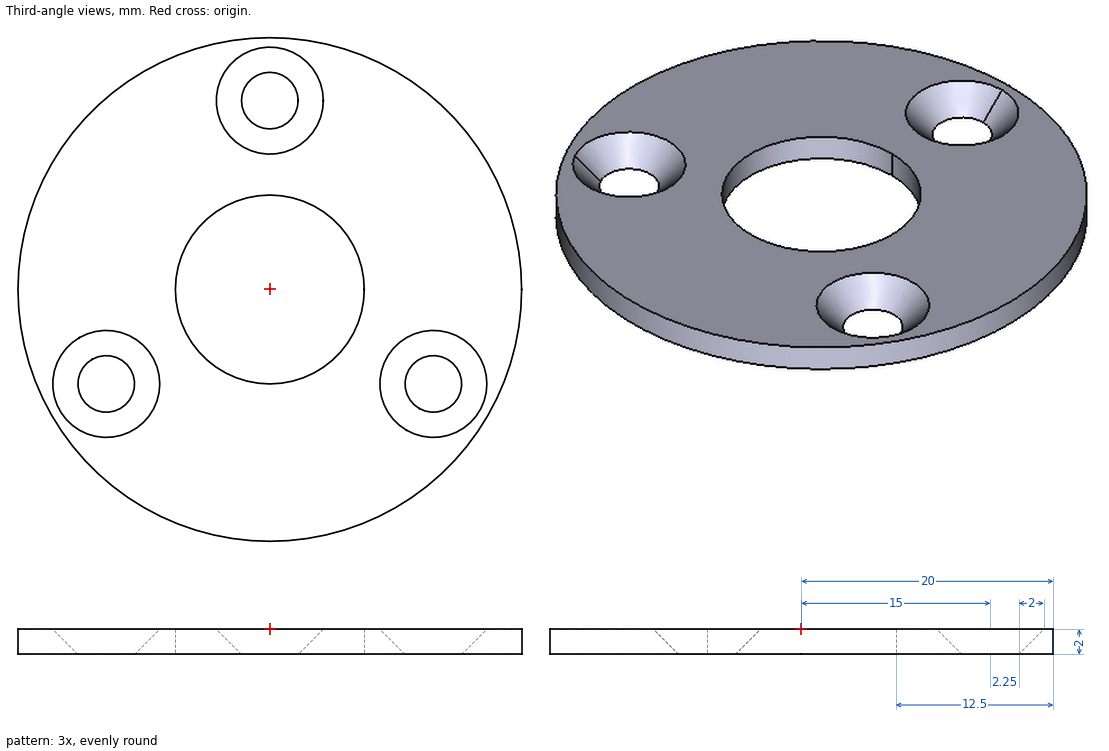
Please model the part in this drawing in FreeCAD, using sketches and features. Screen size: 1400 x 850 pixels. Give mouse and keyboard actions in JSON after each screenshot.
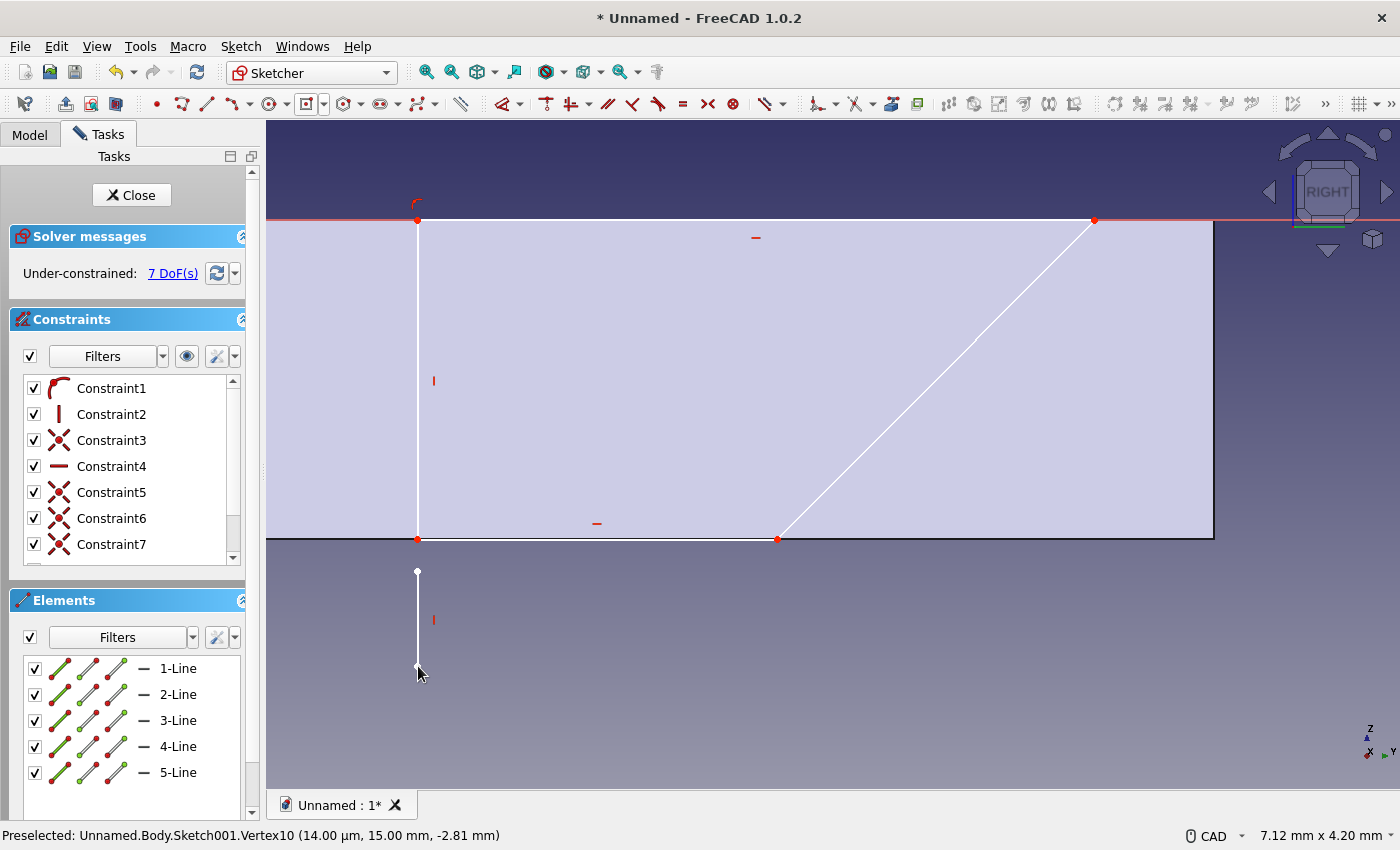
{"action": "left_click", "coordinate": [418, 601]}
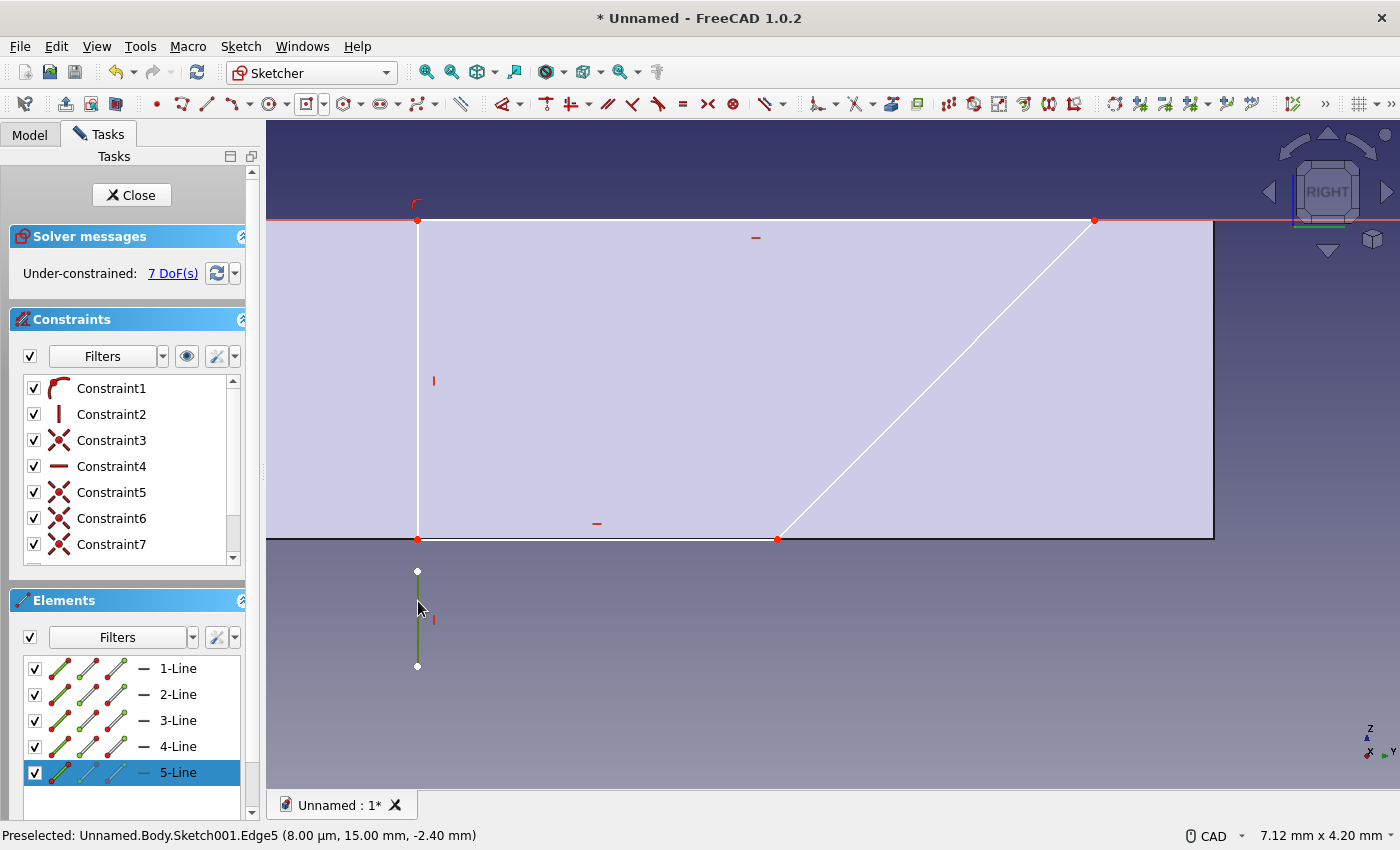
{"action": "left_click", "coordinate": [461, 104]}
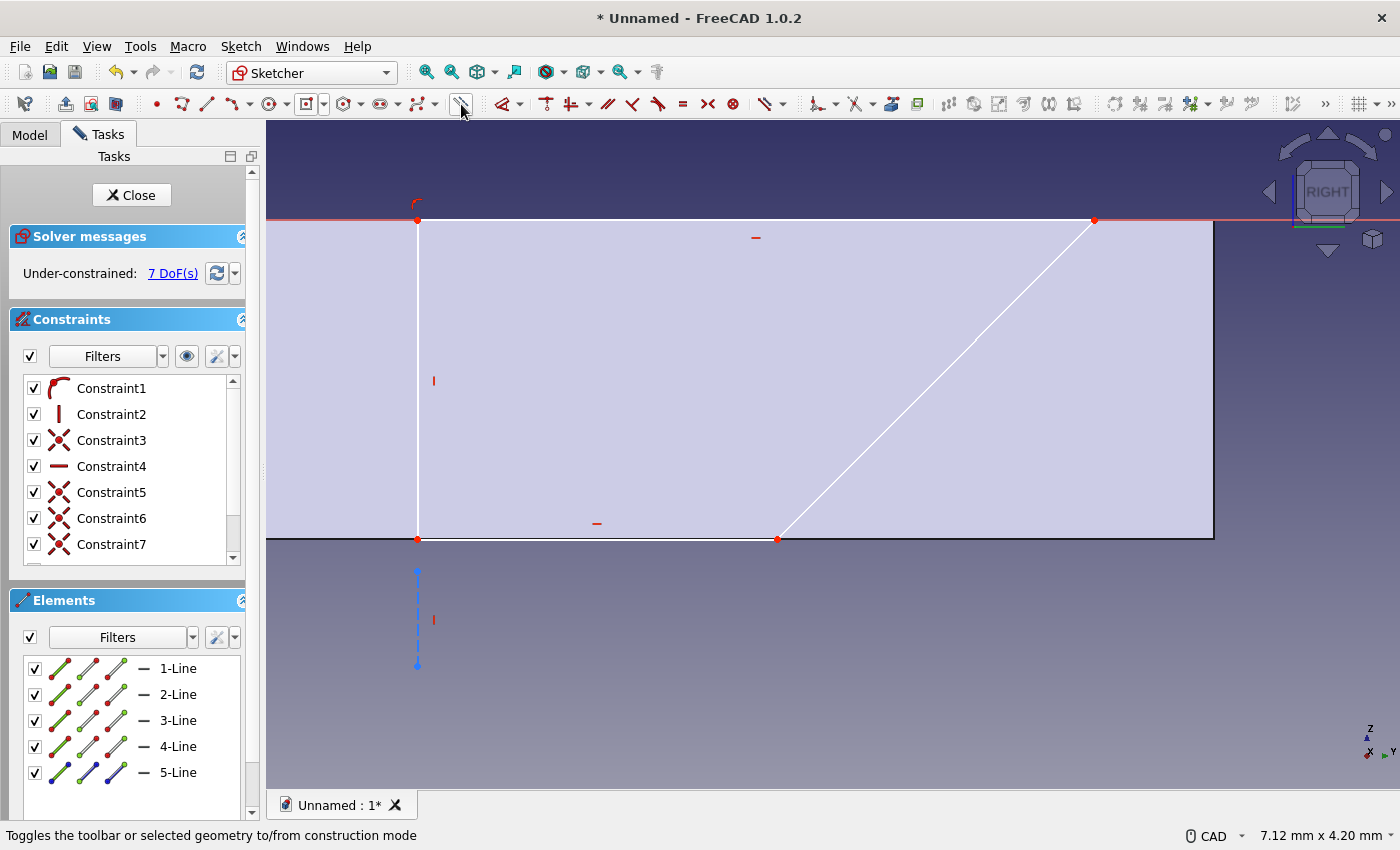
{"action": "left_click", "coordinate": [502, 104]}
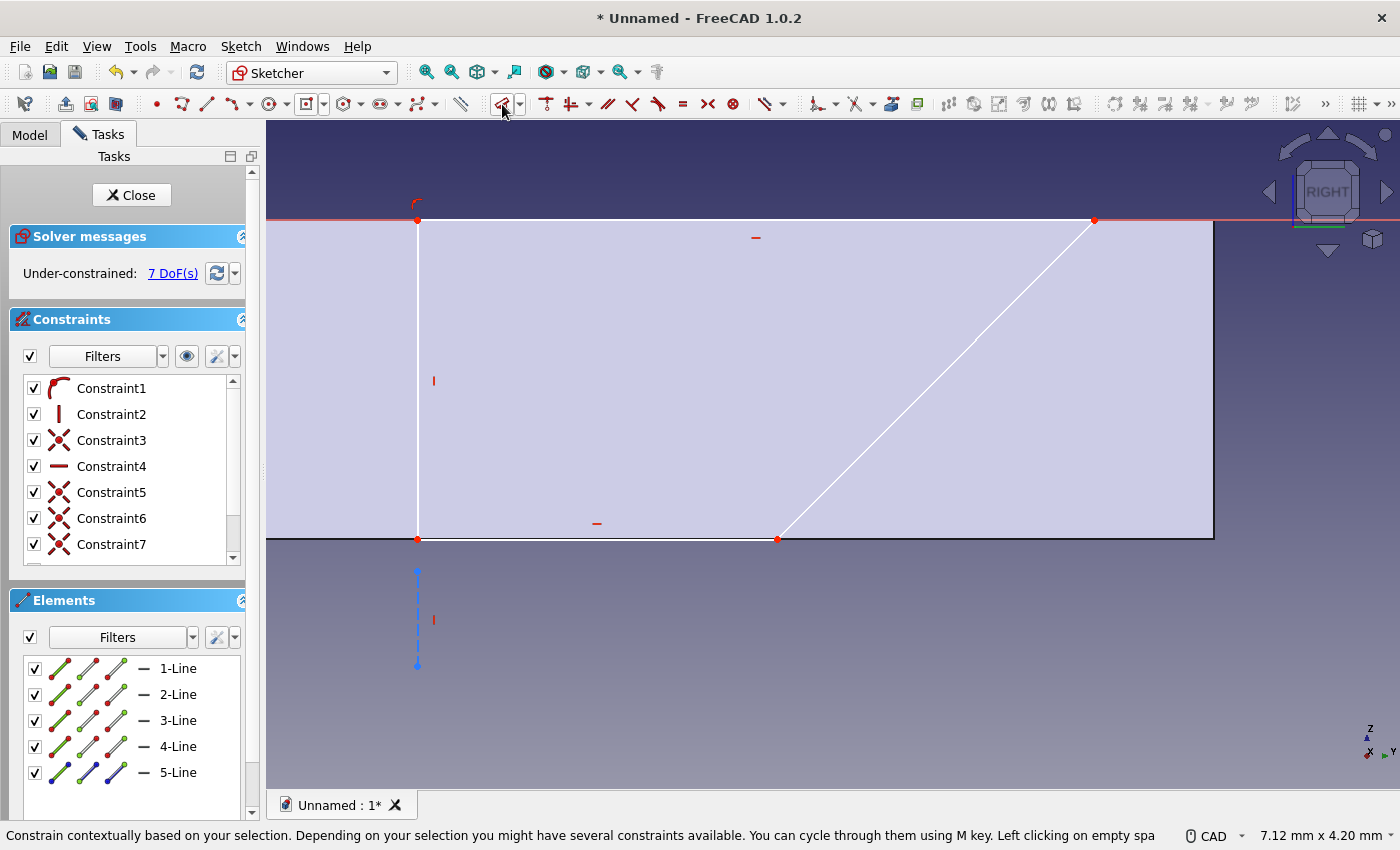
{"action": "left_click", "coordinate": [418, 316]}
{"action": "left_click", "coordinate": [384, 380]}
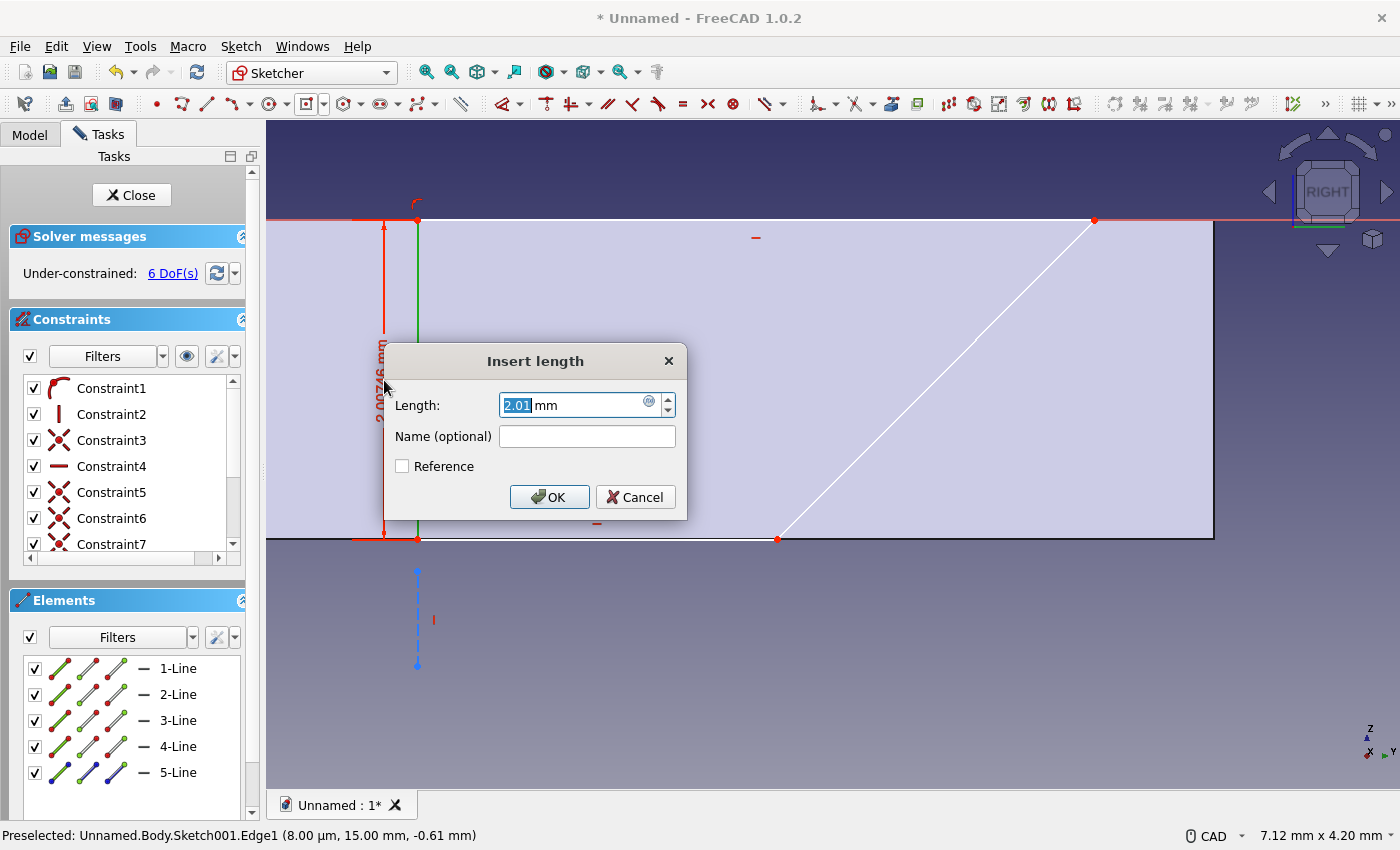
{"action": "type", "text": "2"}
{"action": "key", "text": "Return"}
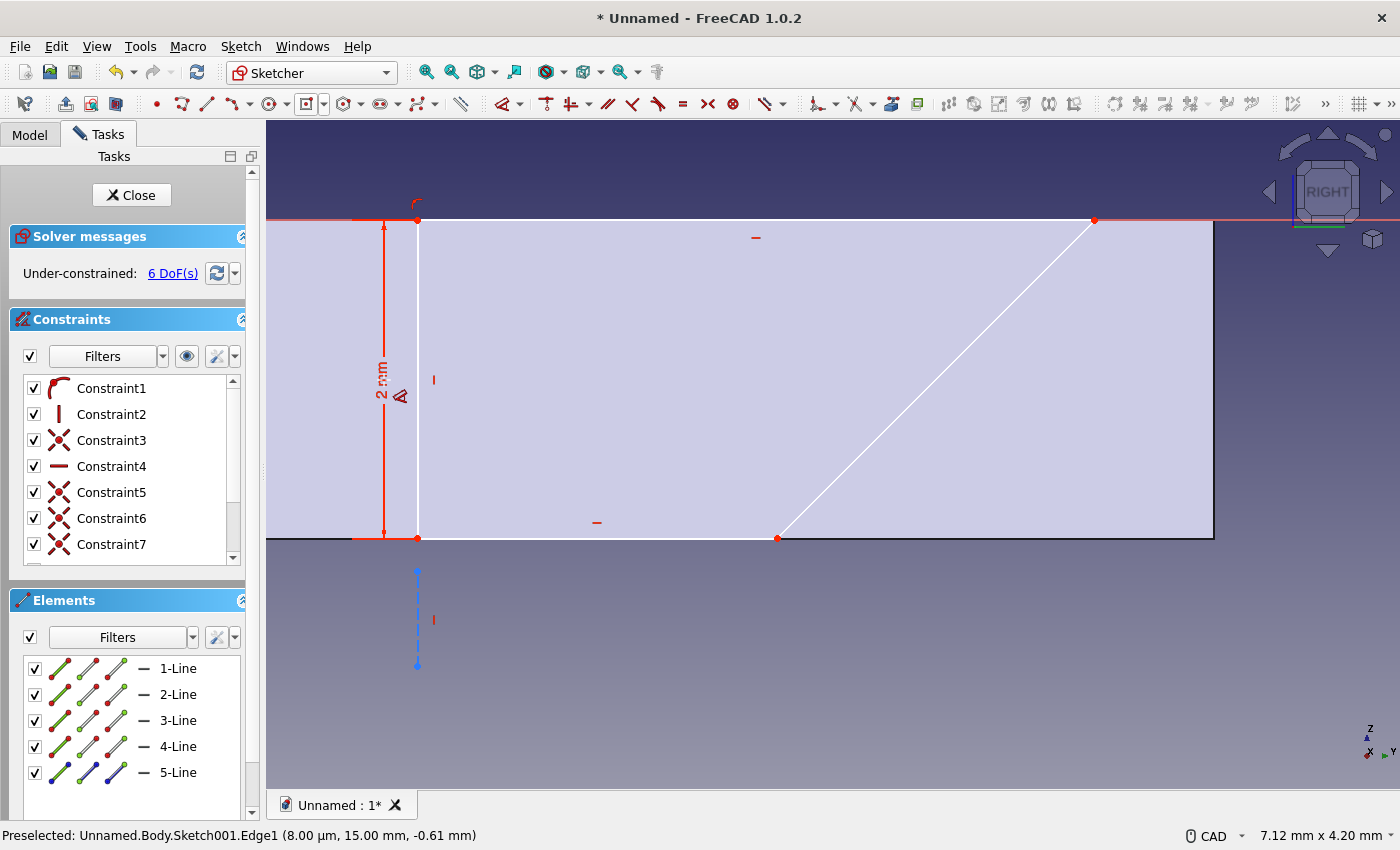
{"action": "left_click", "coordinate": [872, 443]}
{"action": "left_click", "coordinate": [936, 186]}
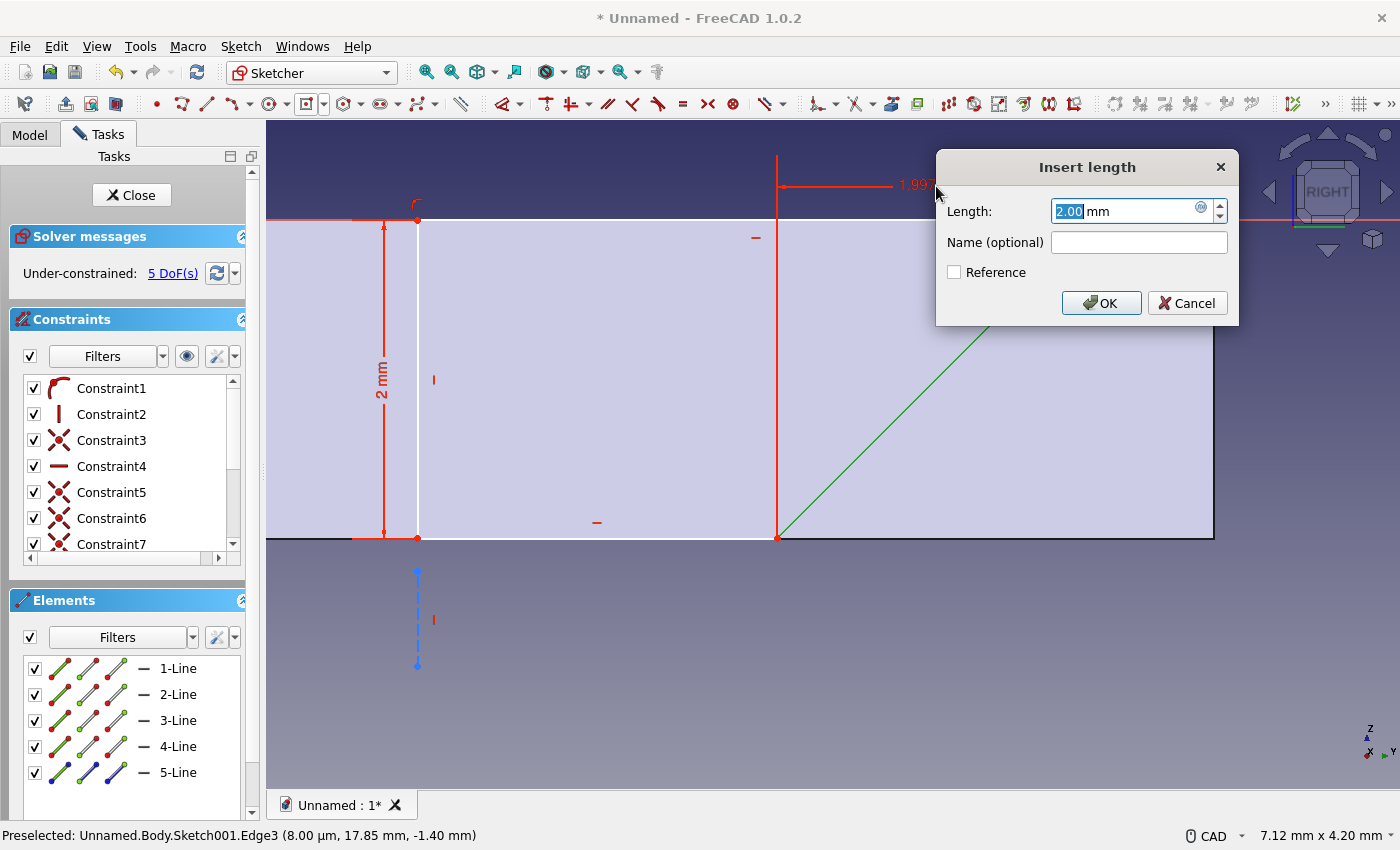
{"action": "type", "text": "2"}
{"action": "key", "text": "Return"}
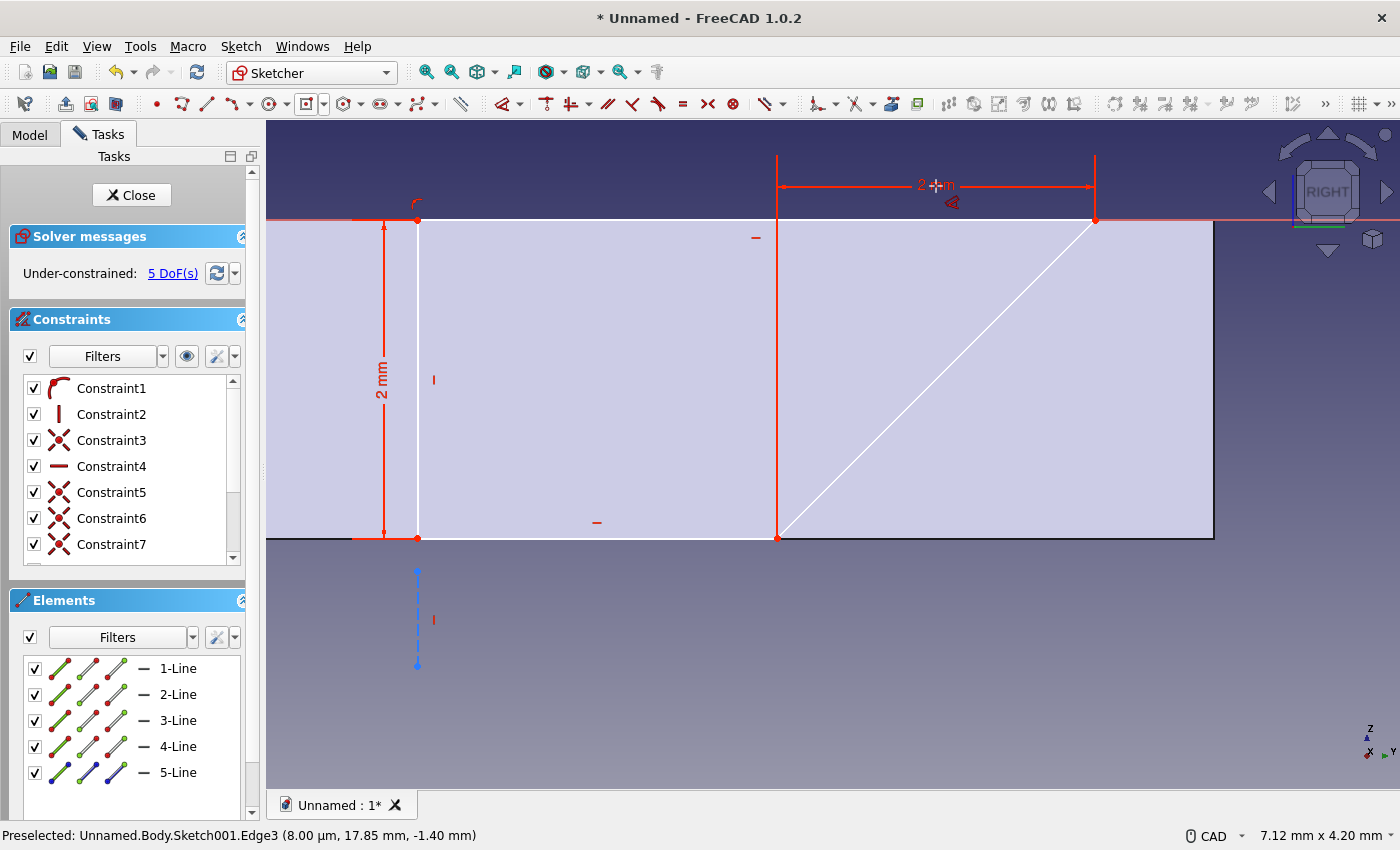
{"action": "left_click", "coordinate": [418, 220]}
{"action": "left_click", "coordinate": [356, 186]}